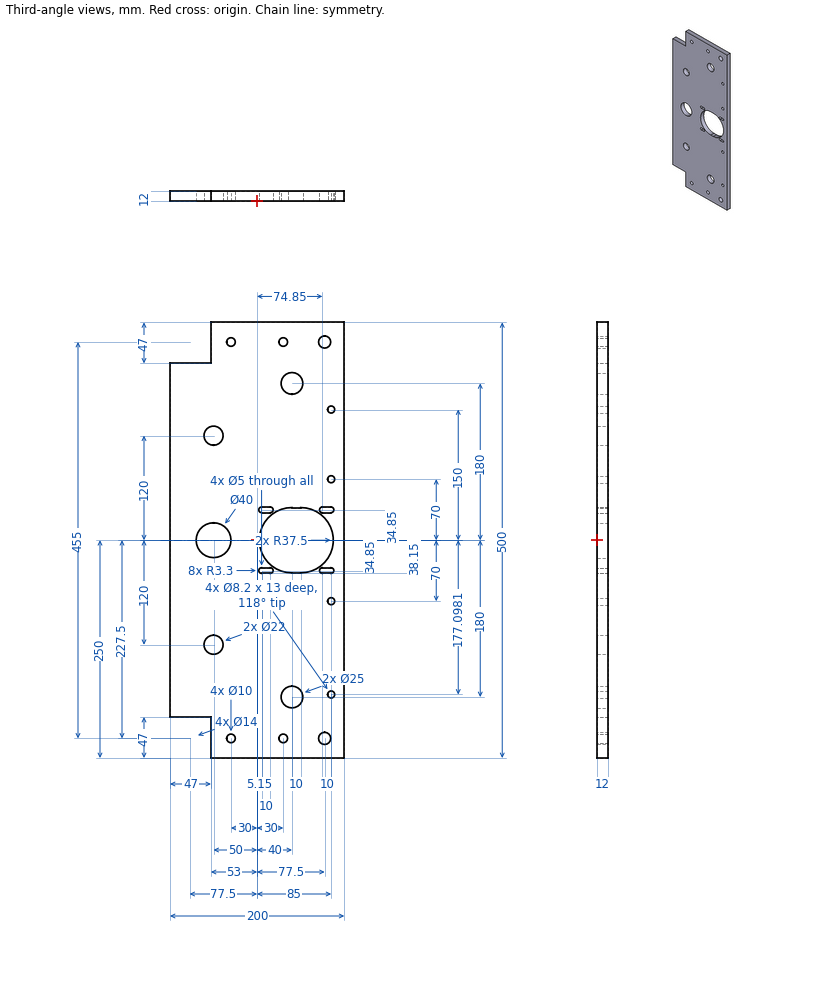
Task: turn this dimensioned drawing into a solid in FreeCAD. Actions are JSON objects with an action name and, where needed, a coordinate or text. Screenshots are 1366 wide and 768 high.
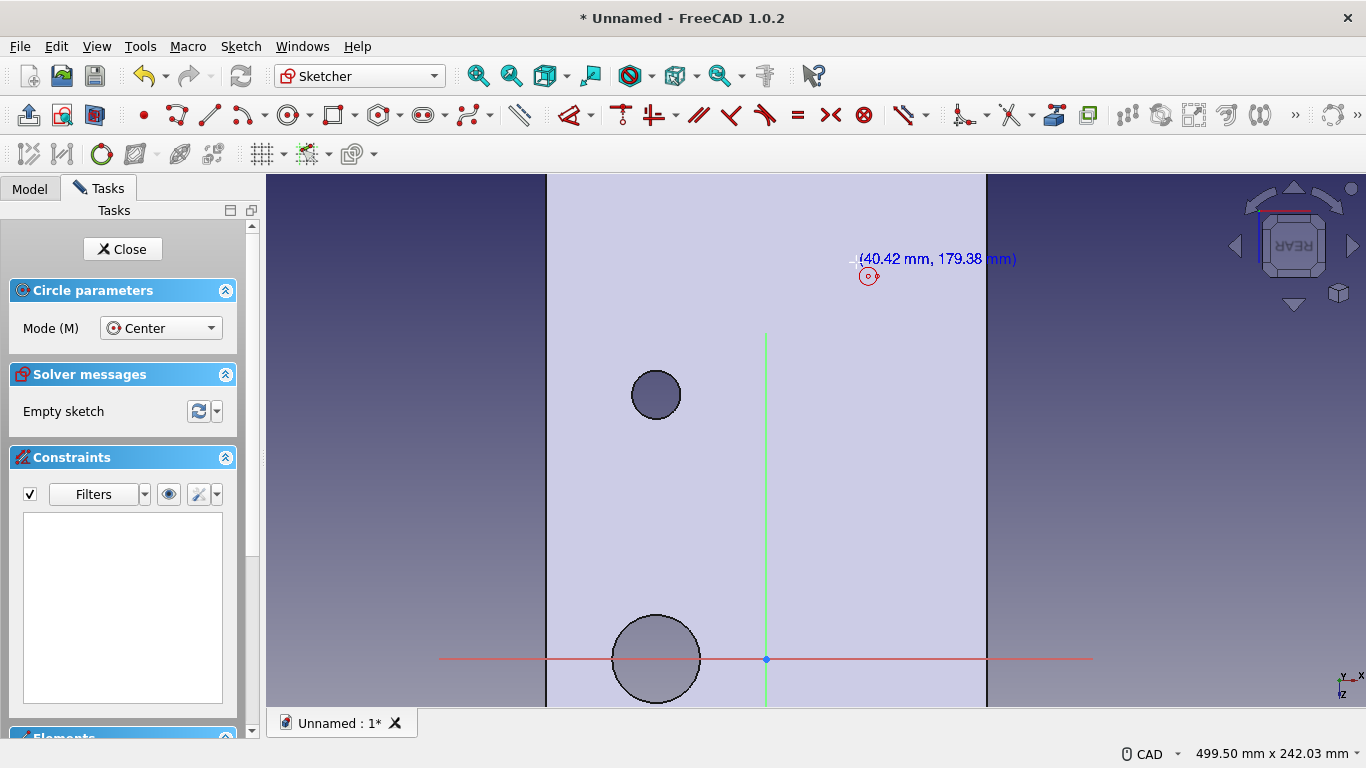
{"action": "left_click", "coordinate": [854, 263]}
{"action": "mouse_move", "coordinate": [874, 243]}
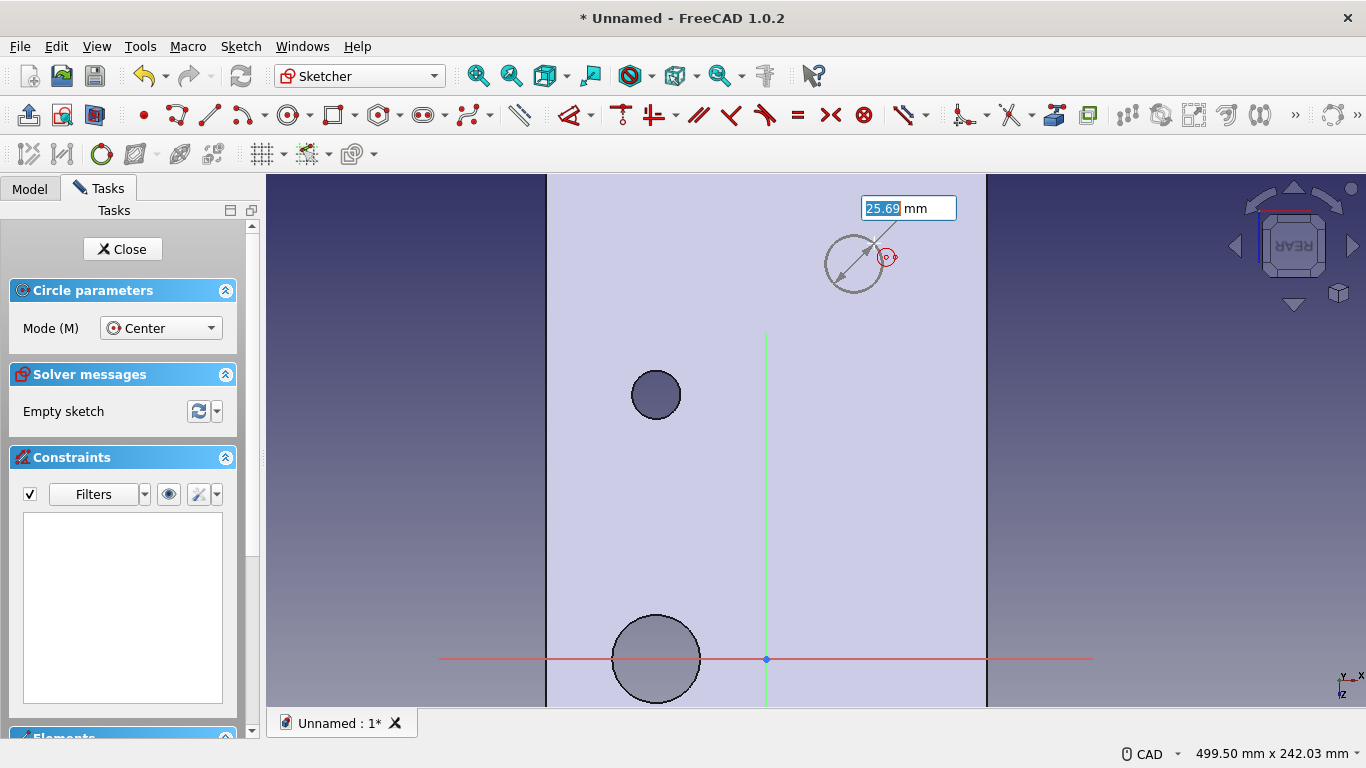
{"action": "type", "text": "25"}
{"action": "key", "text": "Return"}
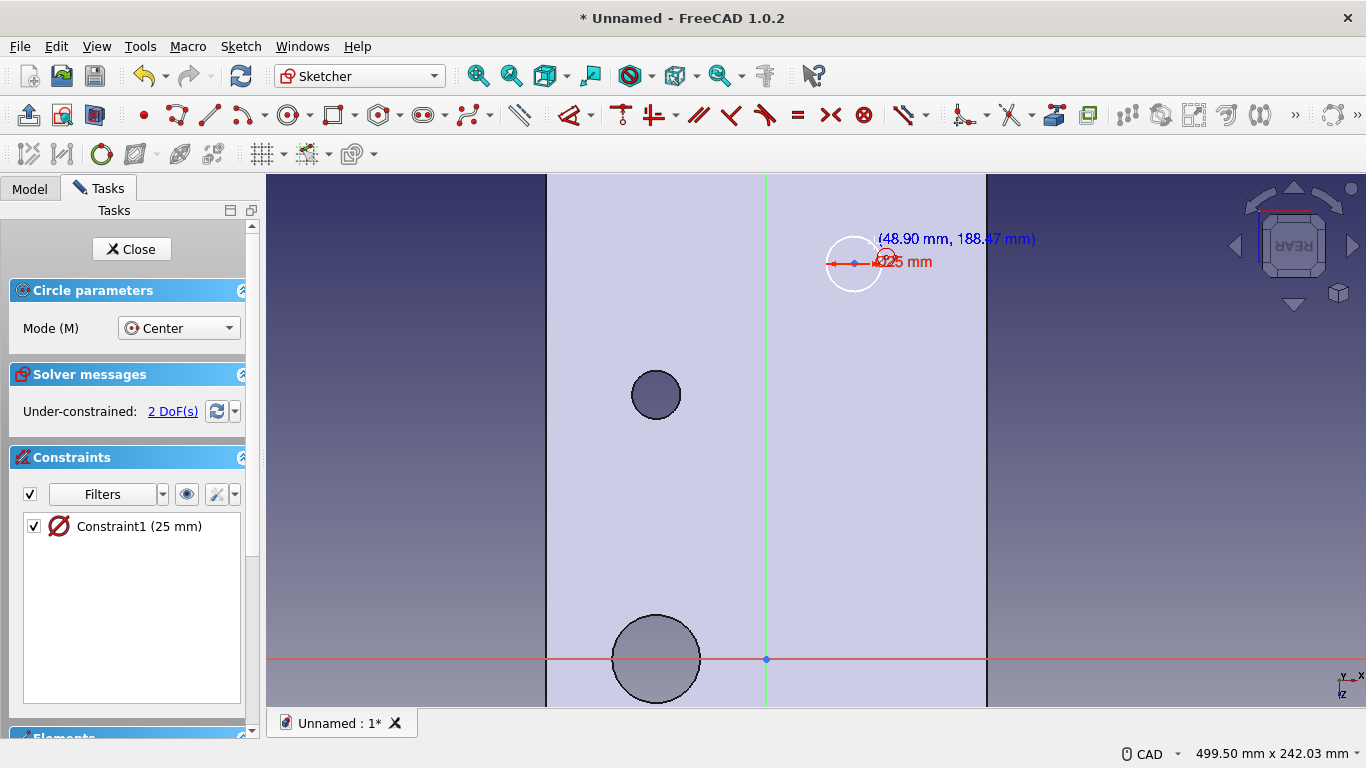
{"action": "scroll", "coordinate": [703, 313], "scroll_direction": "down", "scroll_amount": 5}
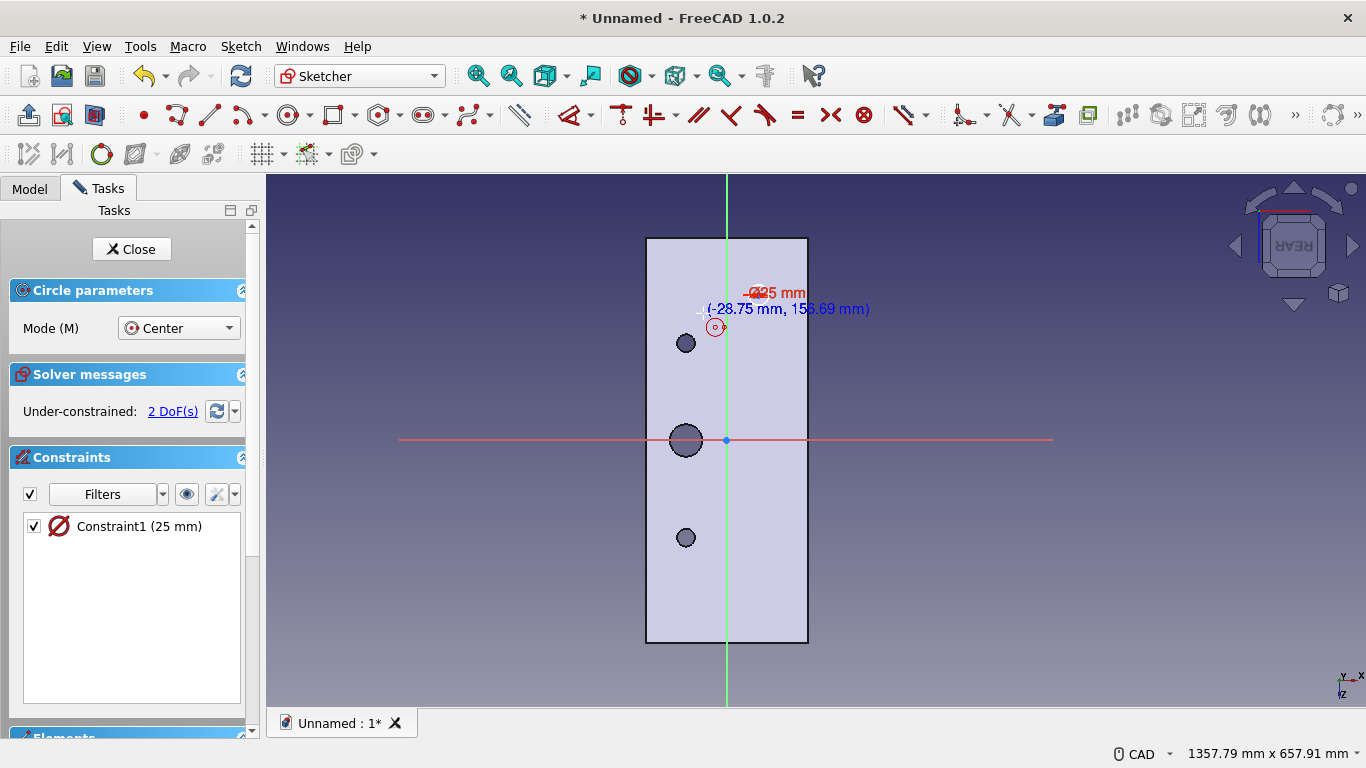
{"action": "scroll", "coordinate": [759, 586], "scroll_direction": "up", "scroll_amount": 5}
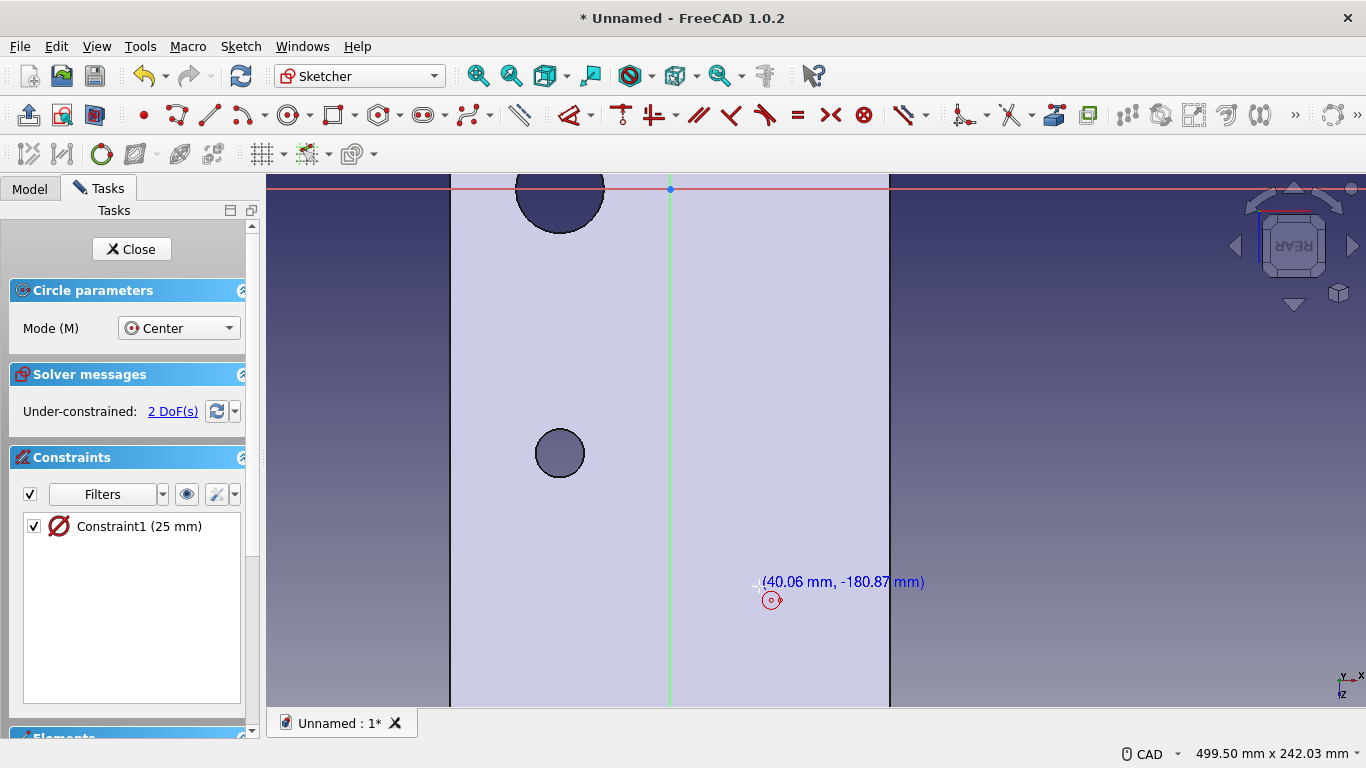
{"action": "left_click", "coordinate": [758, 585]}
{"action": "mouse_move", "coordinate": [778, 566]}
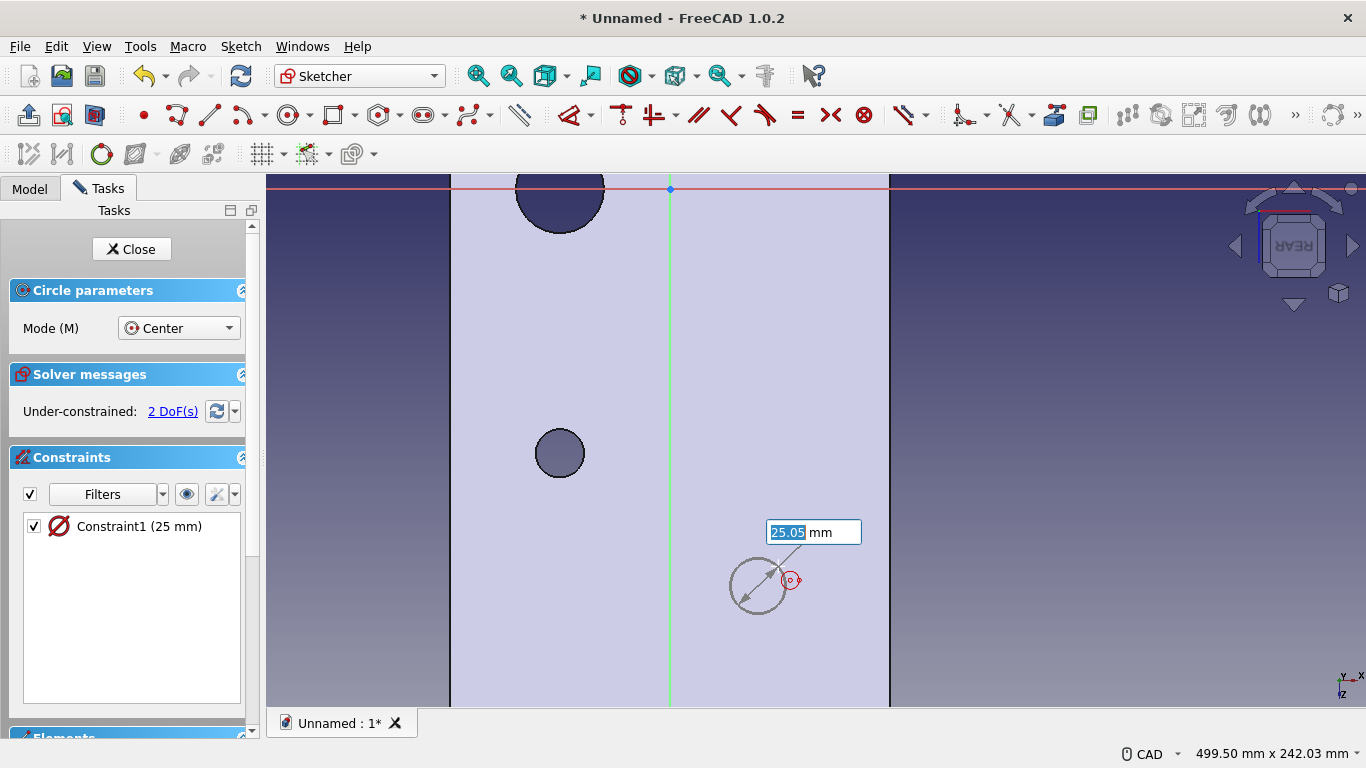
{"action": "type", "text": "25"}
{"action": "key", "text": "Return"}
{"action": "key", "text": "Escape"}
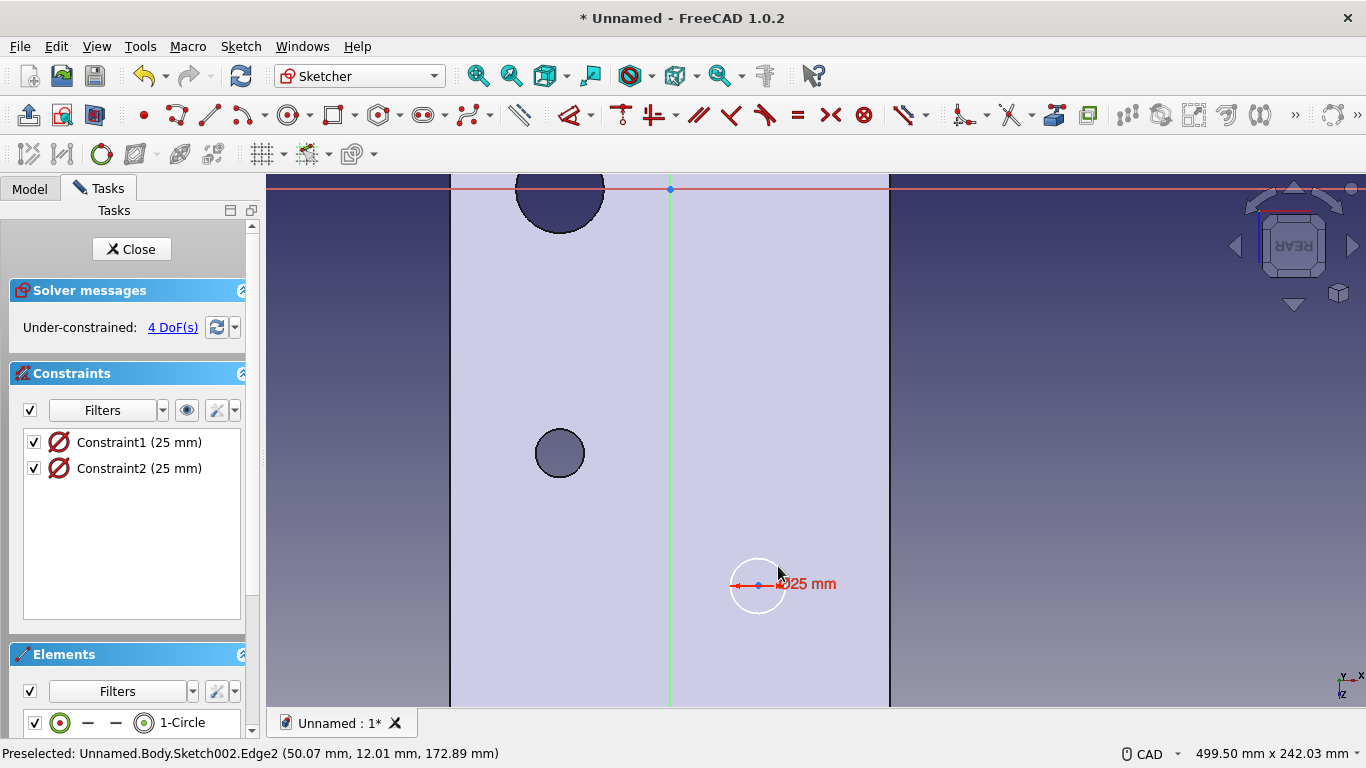
{"action": "scroll", "coordinate": [759, 587], "scroll_direction": "down", "scroll_amount": 5}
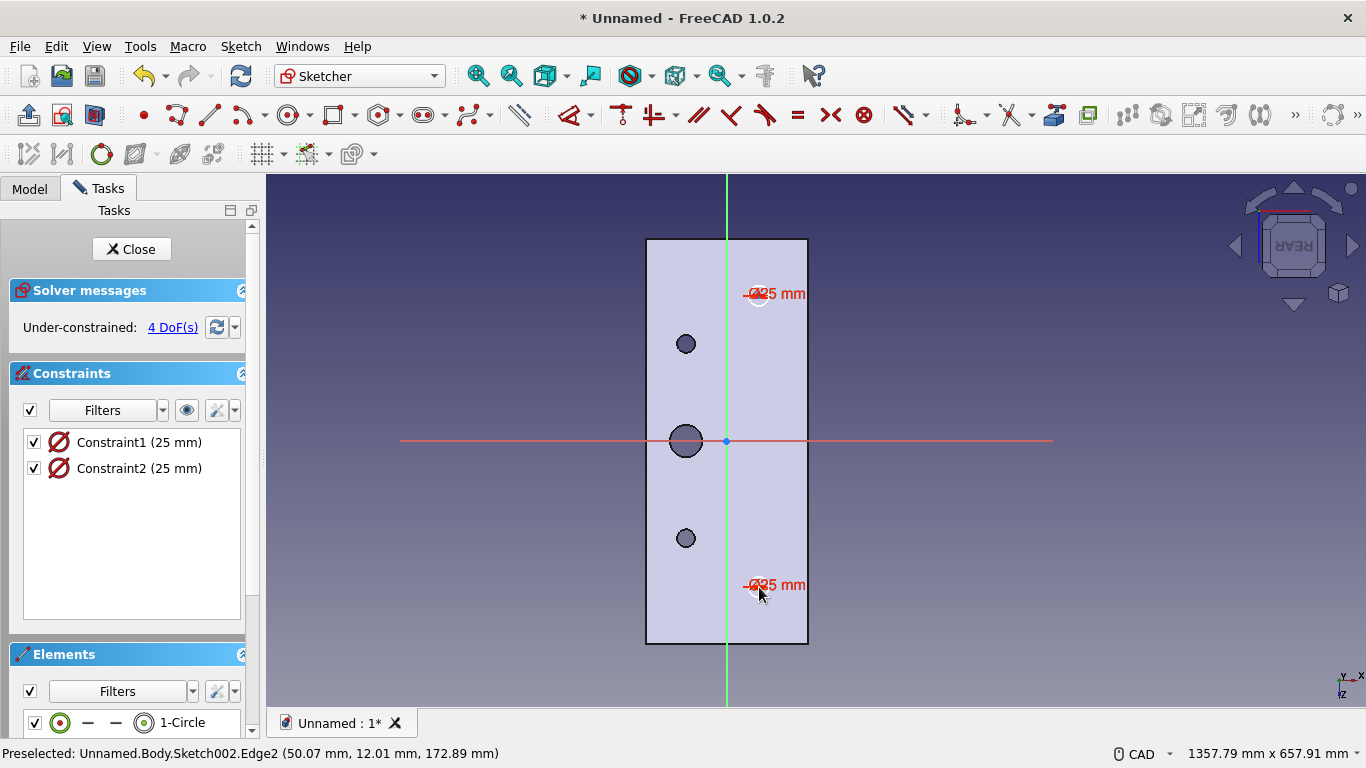
{"action": "left_click", "coordinate": [759, 296]}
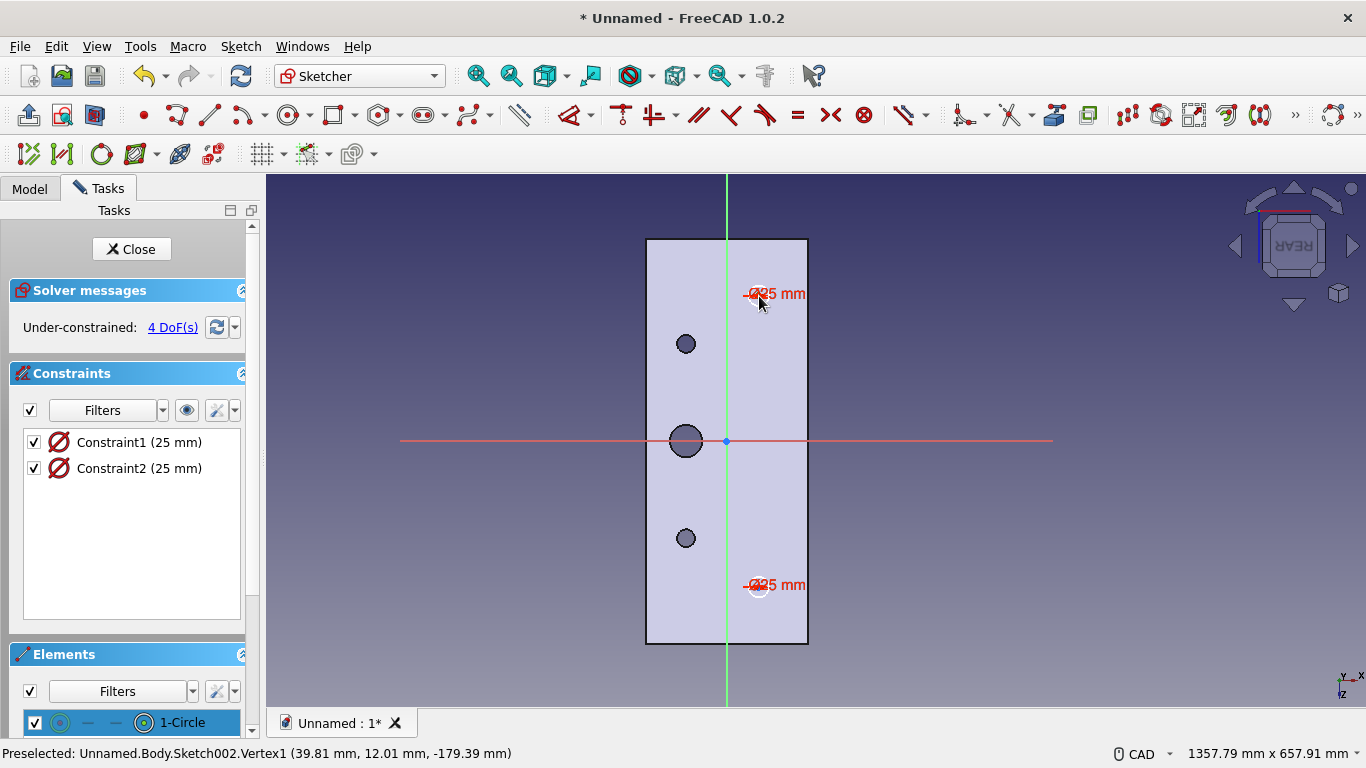
{"action": "left_click", "coordinate": [759, 587]}